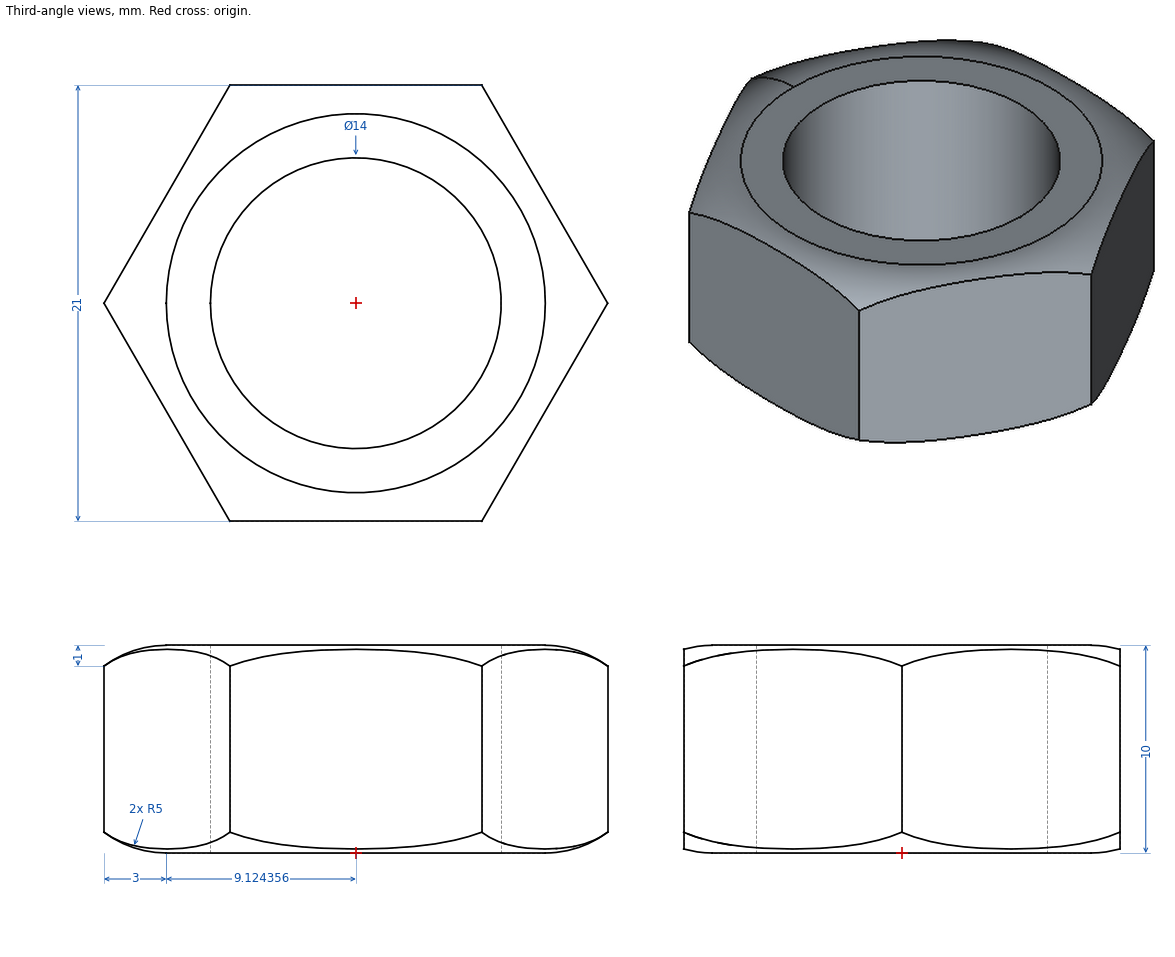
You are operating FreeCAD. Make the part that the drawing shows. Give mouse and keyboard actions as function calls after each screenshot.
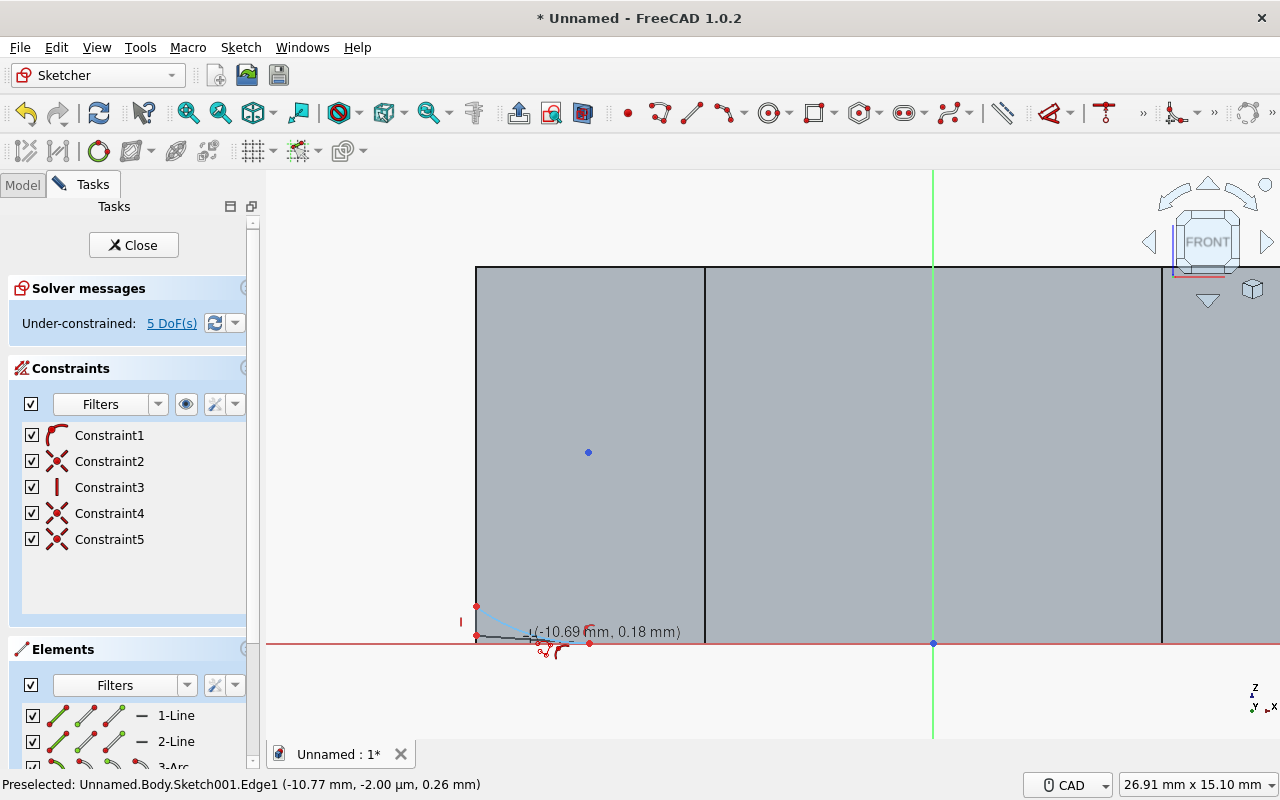
click(476, 304)
click(476, 267)
click(589, 267)
right_click(589, 267)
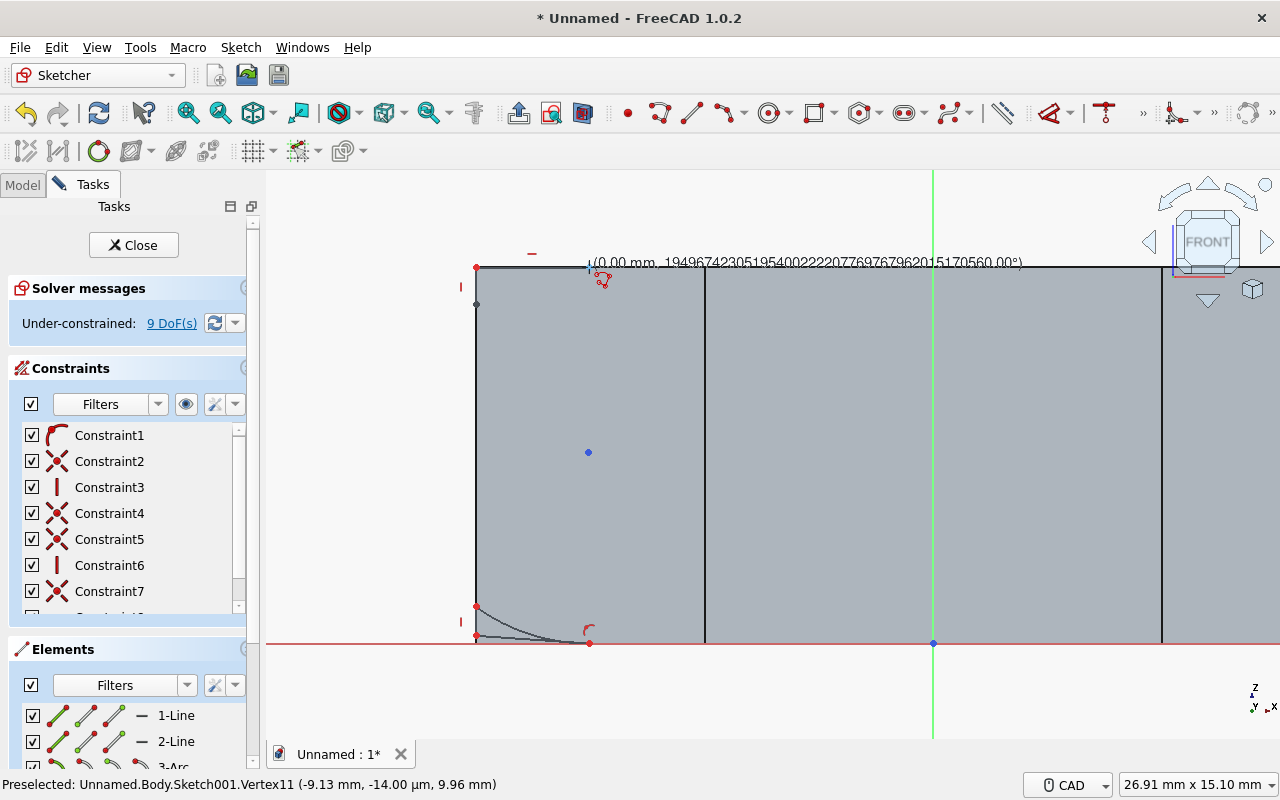
key(g)
key(3)
key(a)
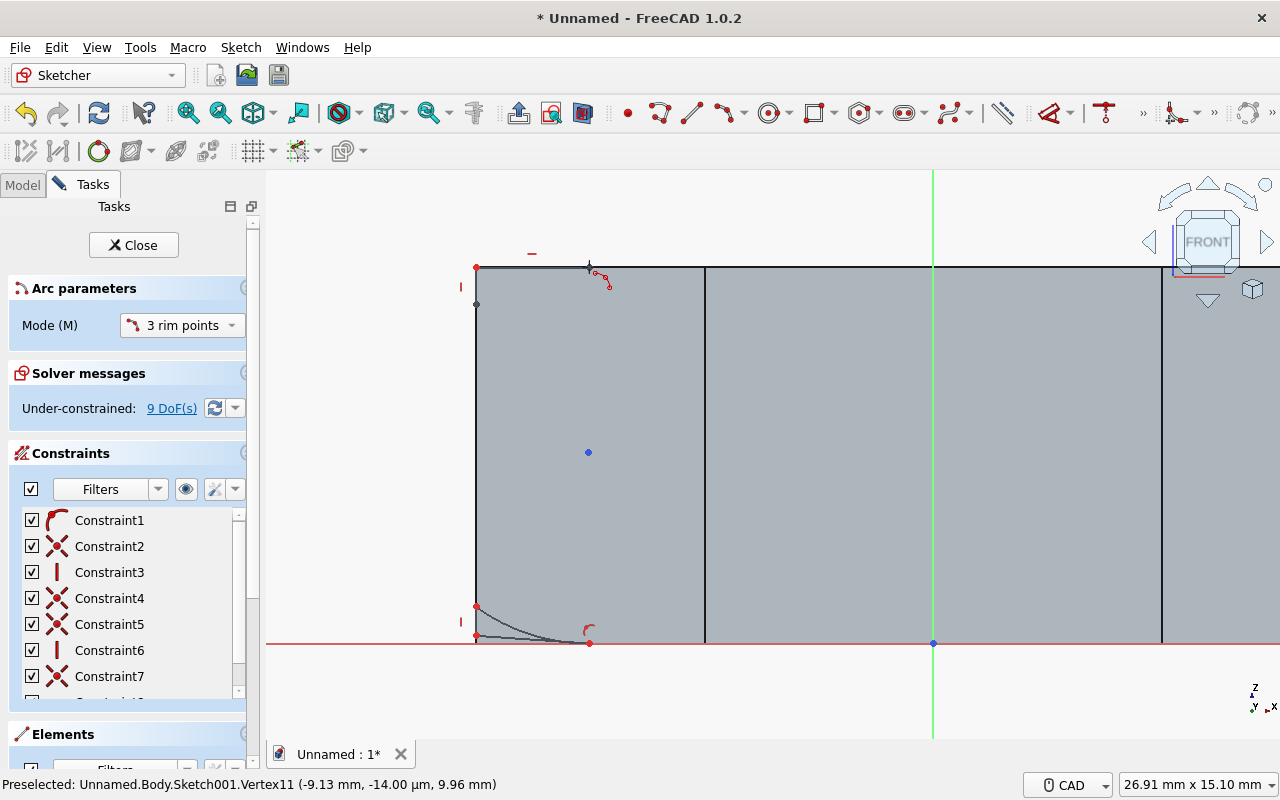
click(589, 268)
click(476, 305)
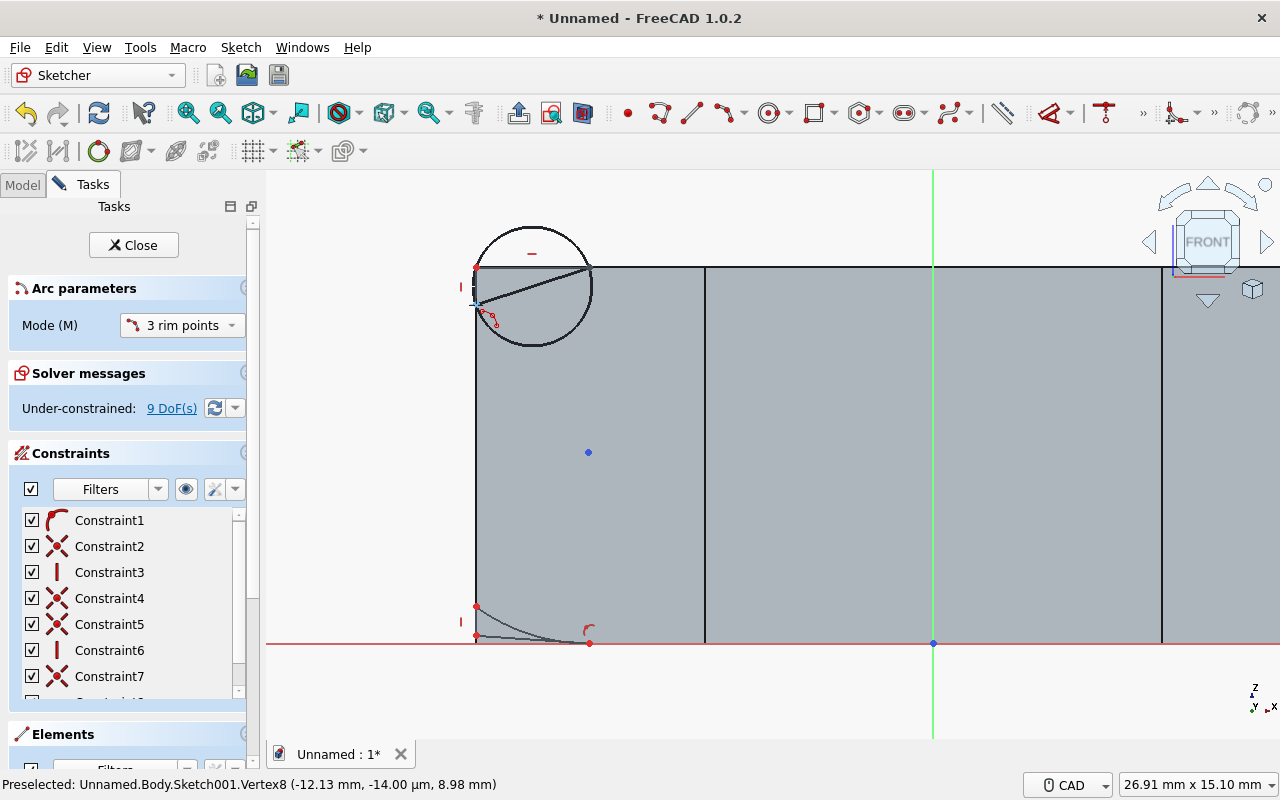
scroll(530, 276, up, 3)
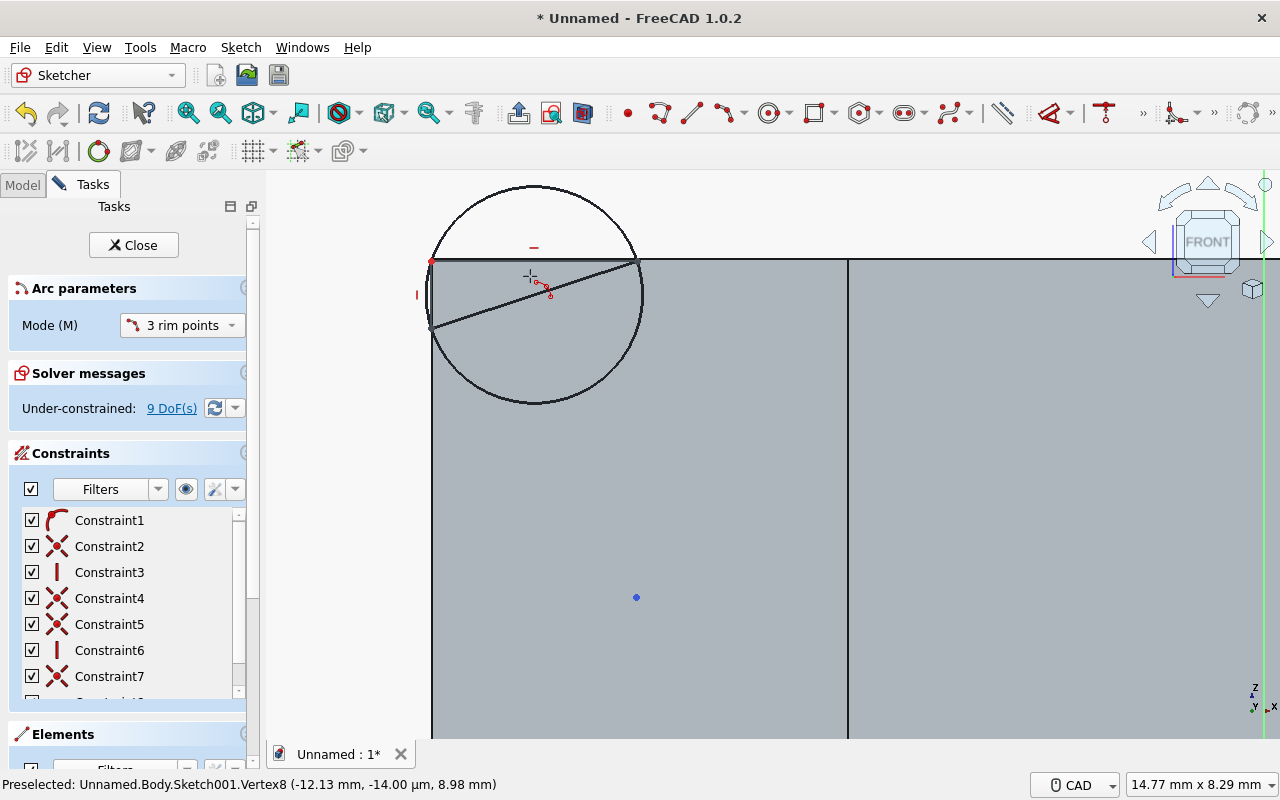
click(529, 276)
key(Escape)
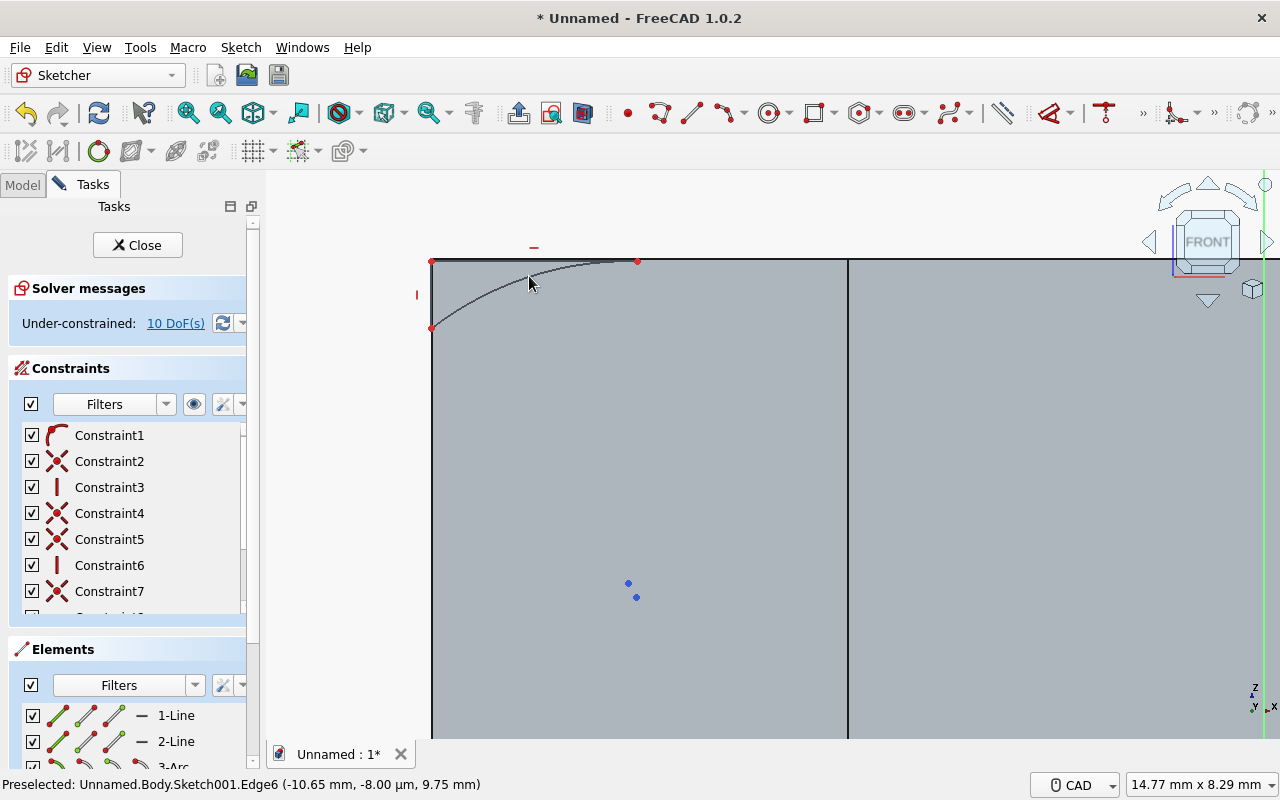
scroll(530, 275, down, 3)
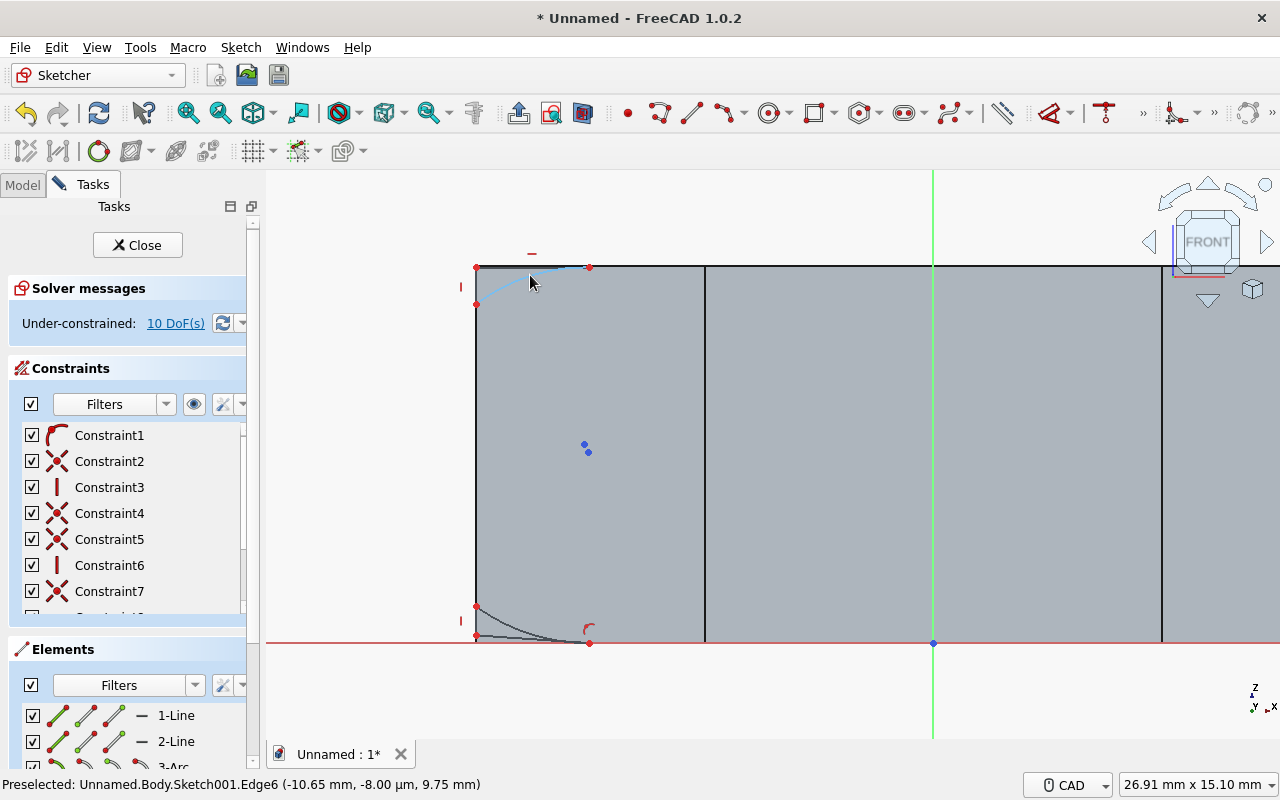
scroll(510, 638, up, 5)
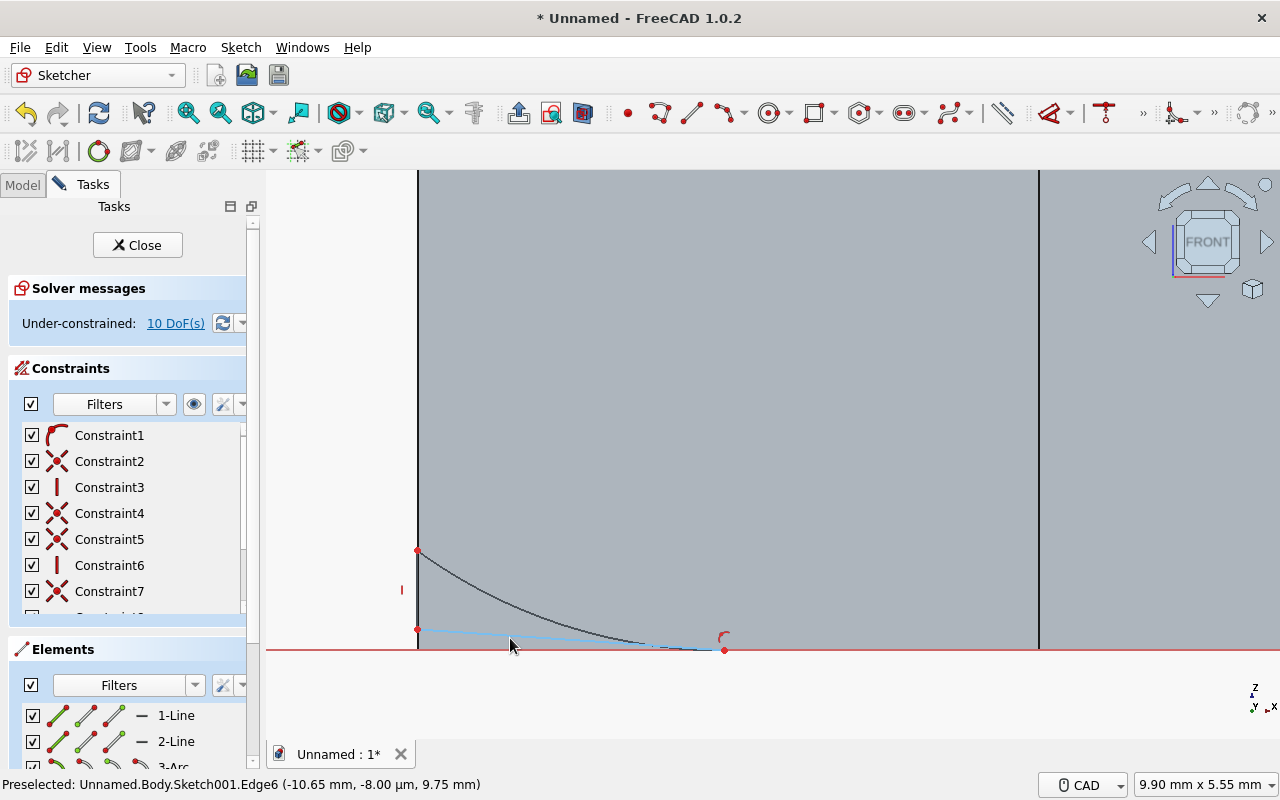
click(509, 636)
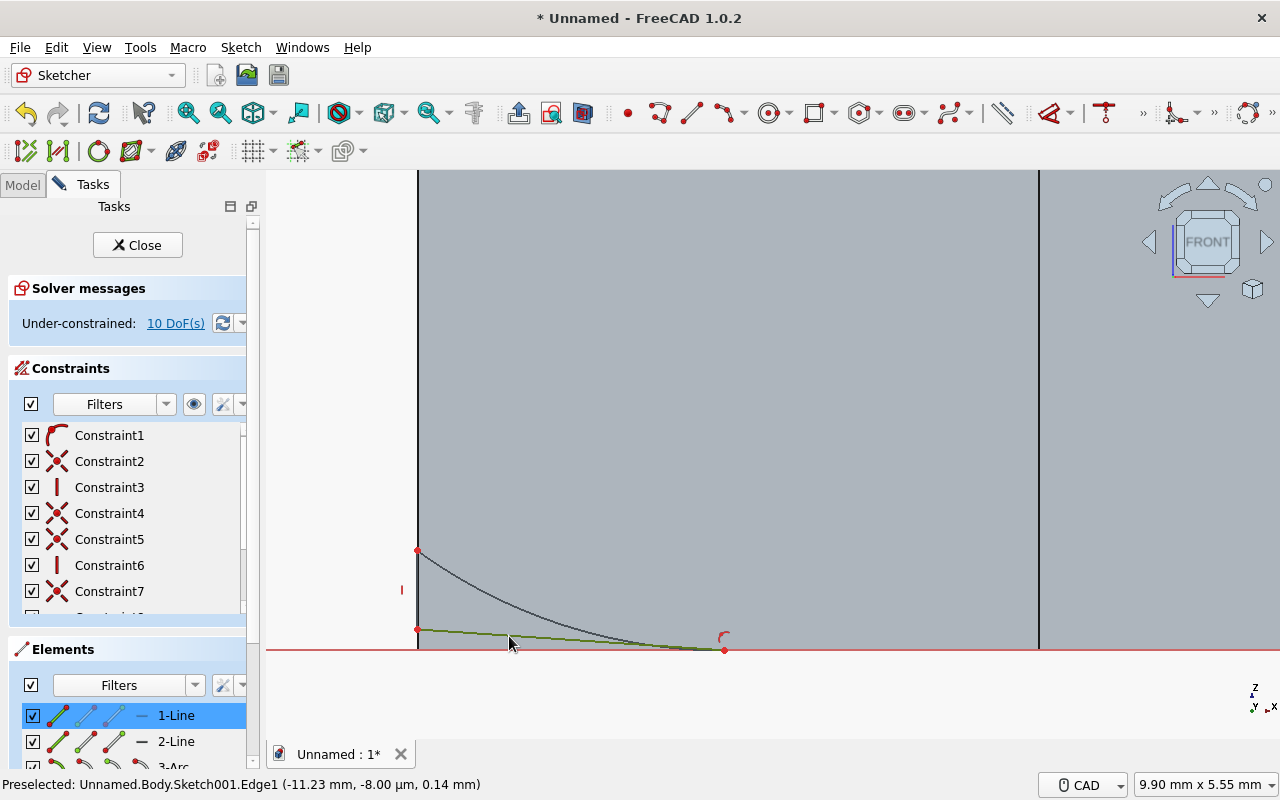
click(502, 601)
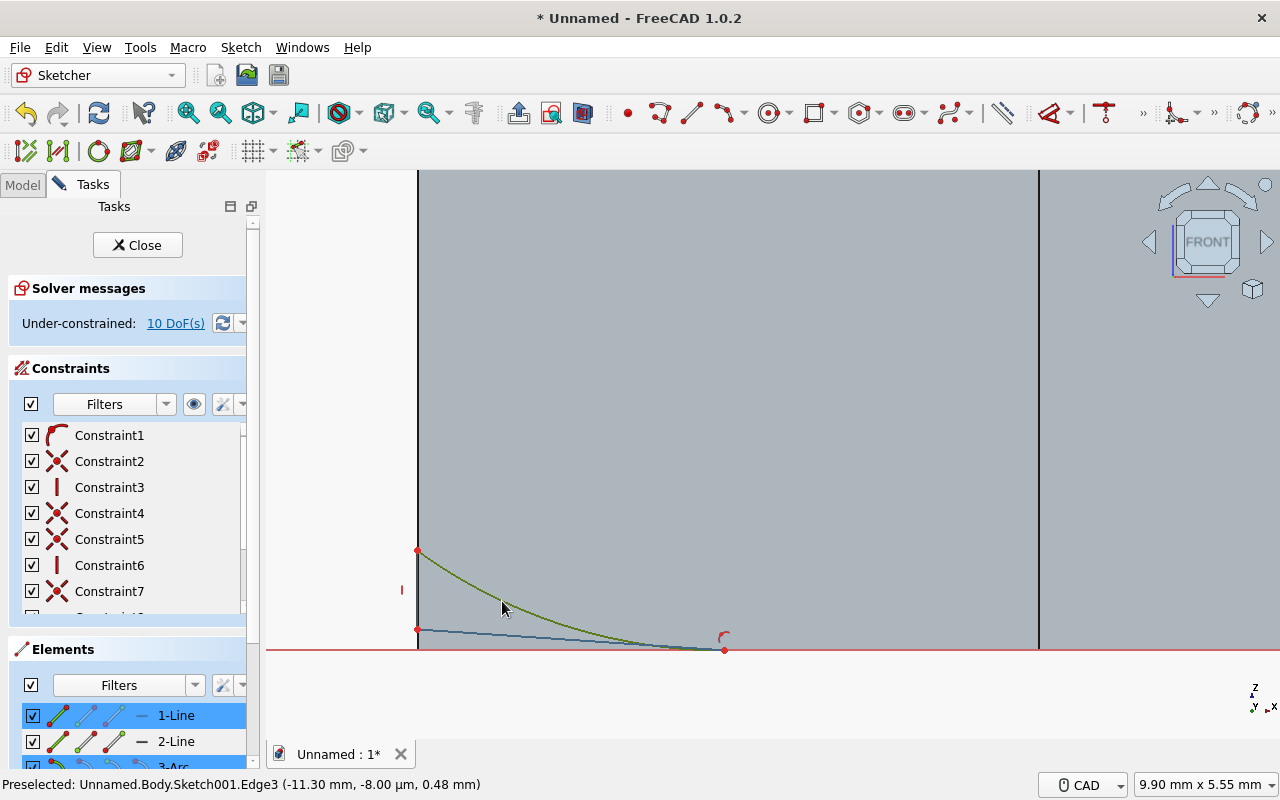
key(t)